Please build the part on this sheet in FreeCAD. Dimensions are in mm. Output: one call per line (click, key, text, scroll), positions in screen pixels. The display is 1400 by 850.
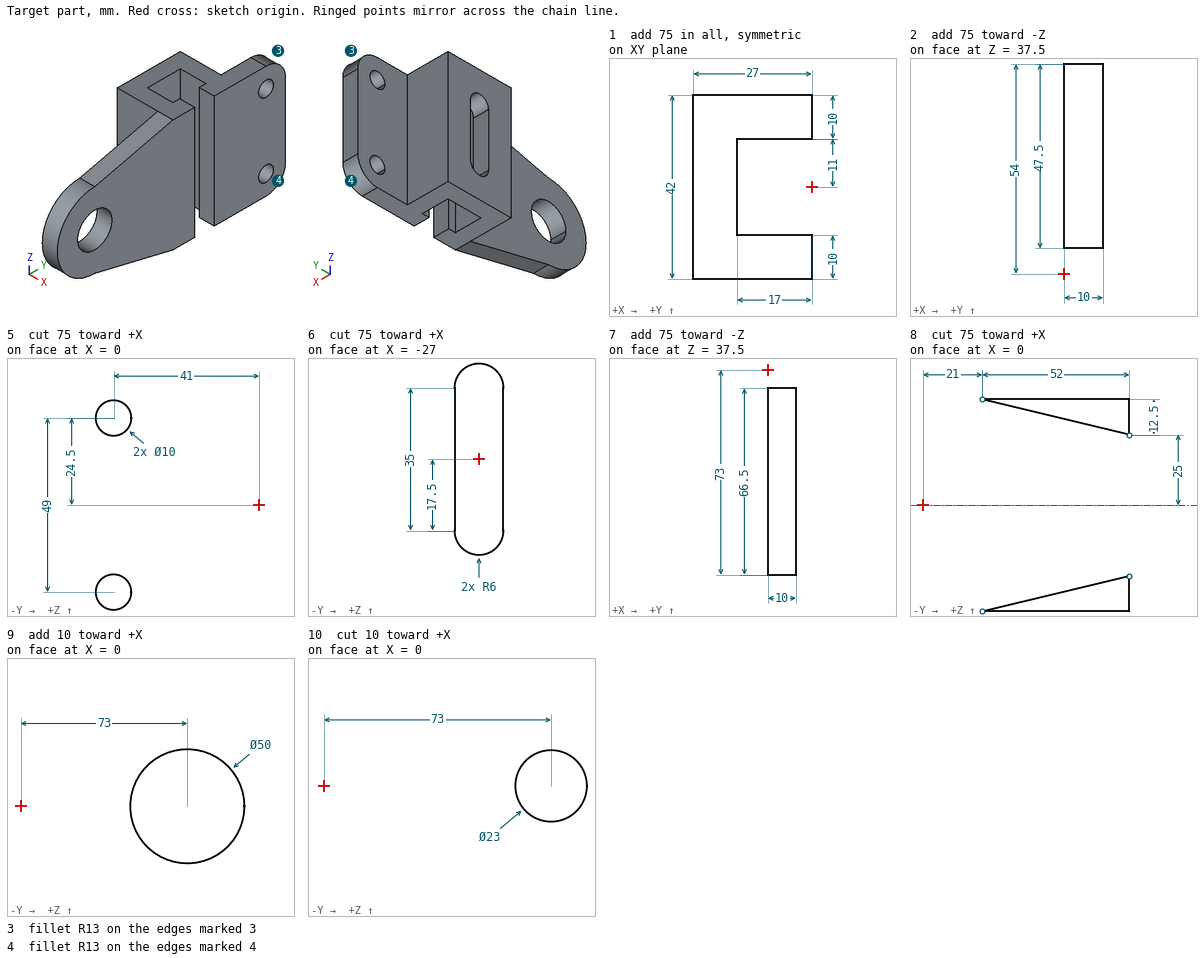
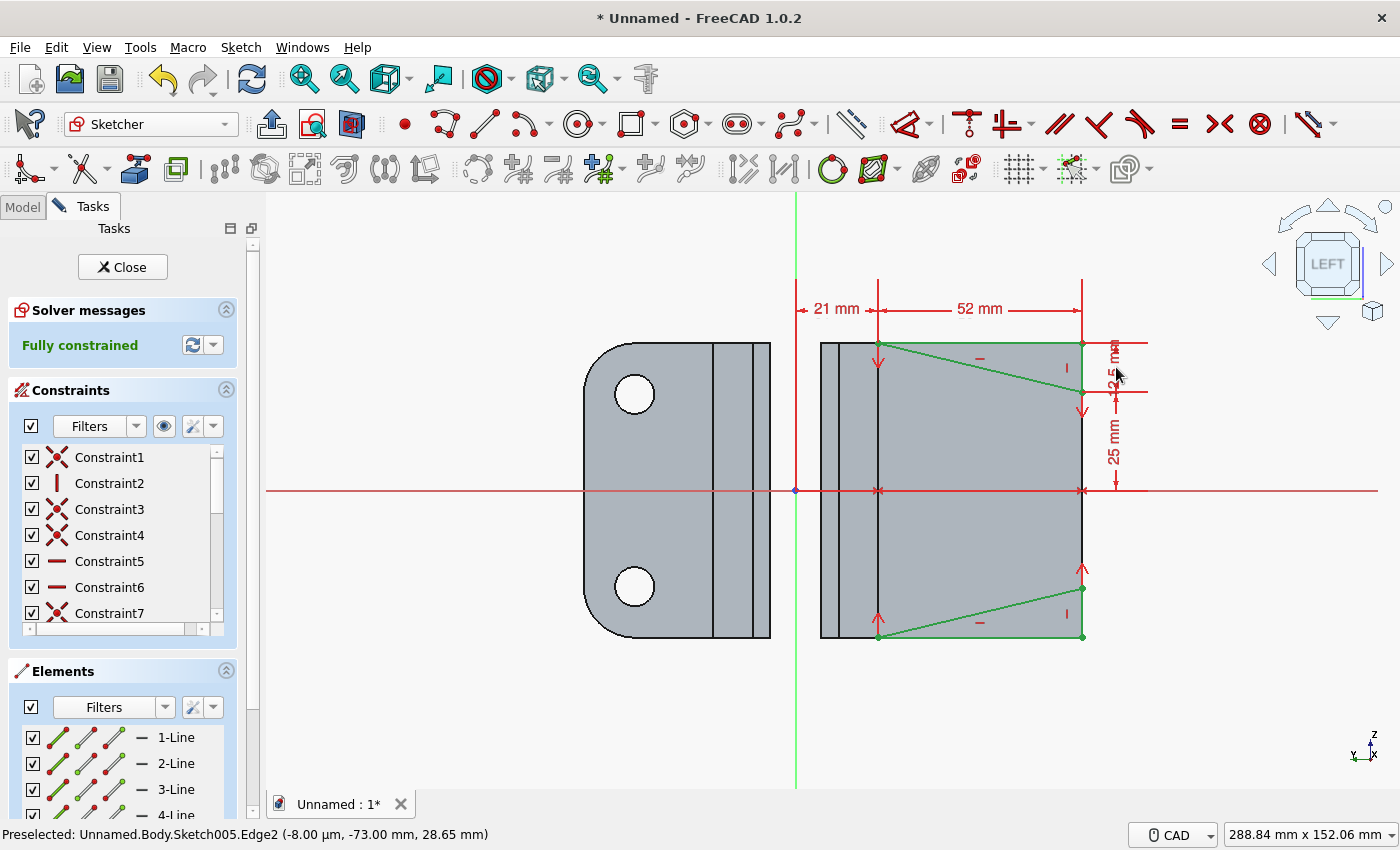
click(123, 267)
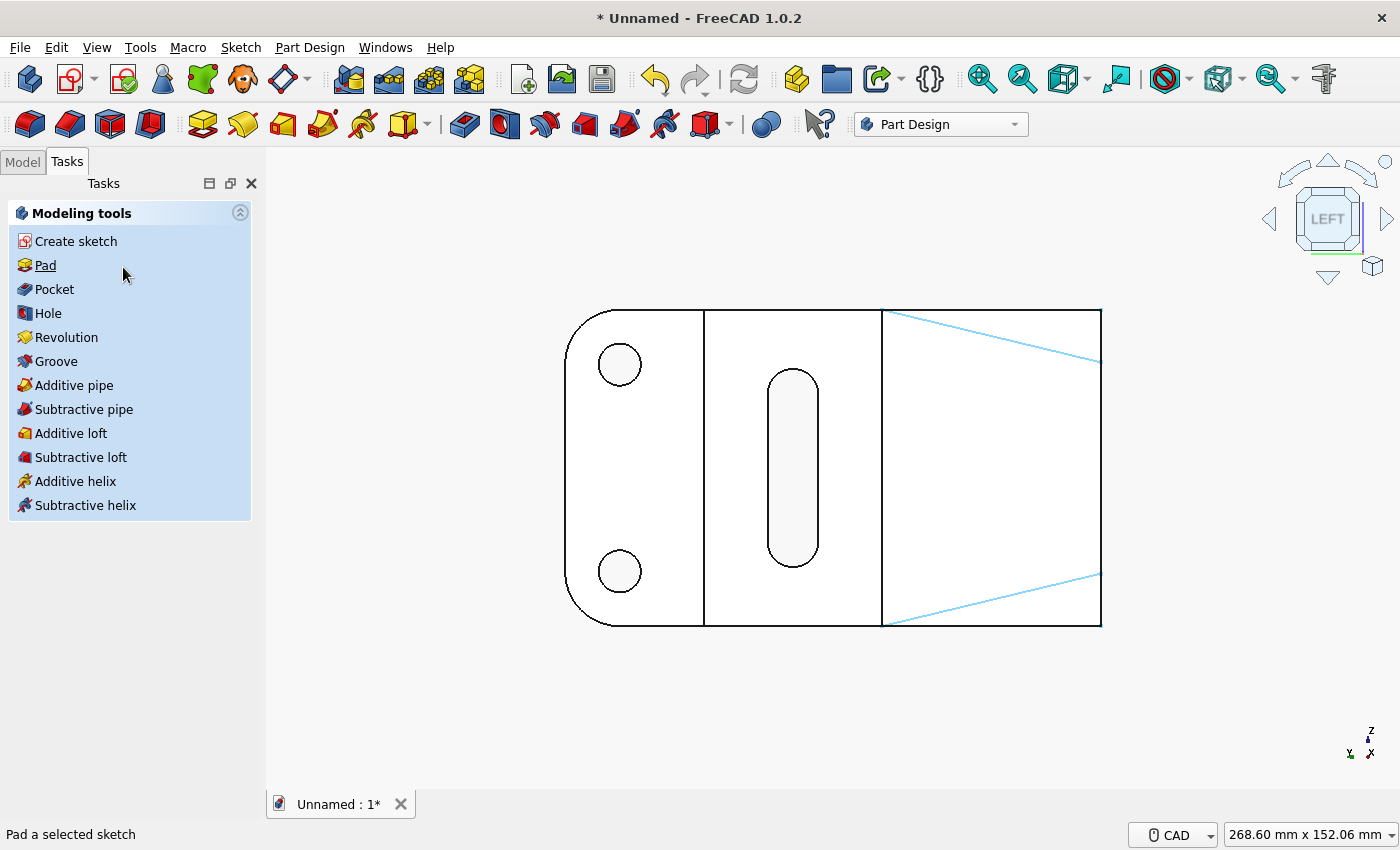
click(466, 124)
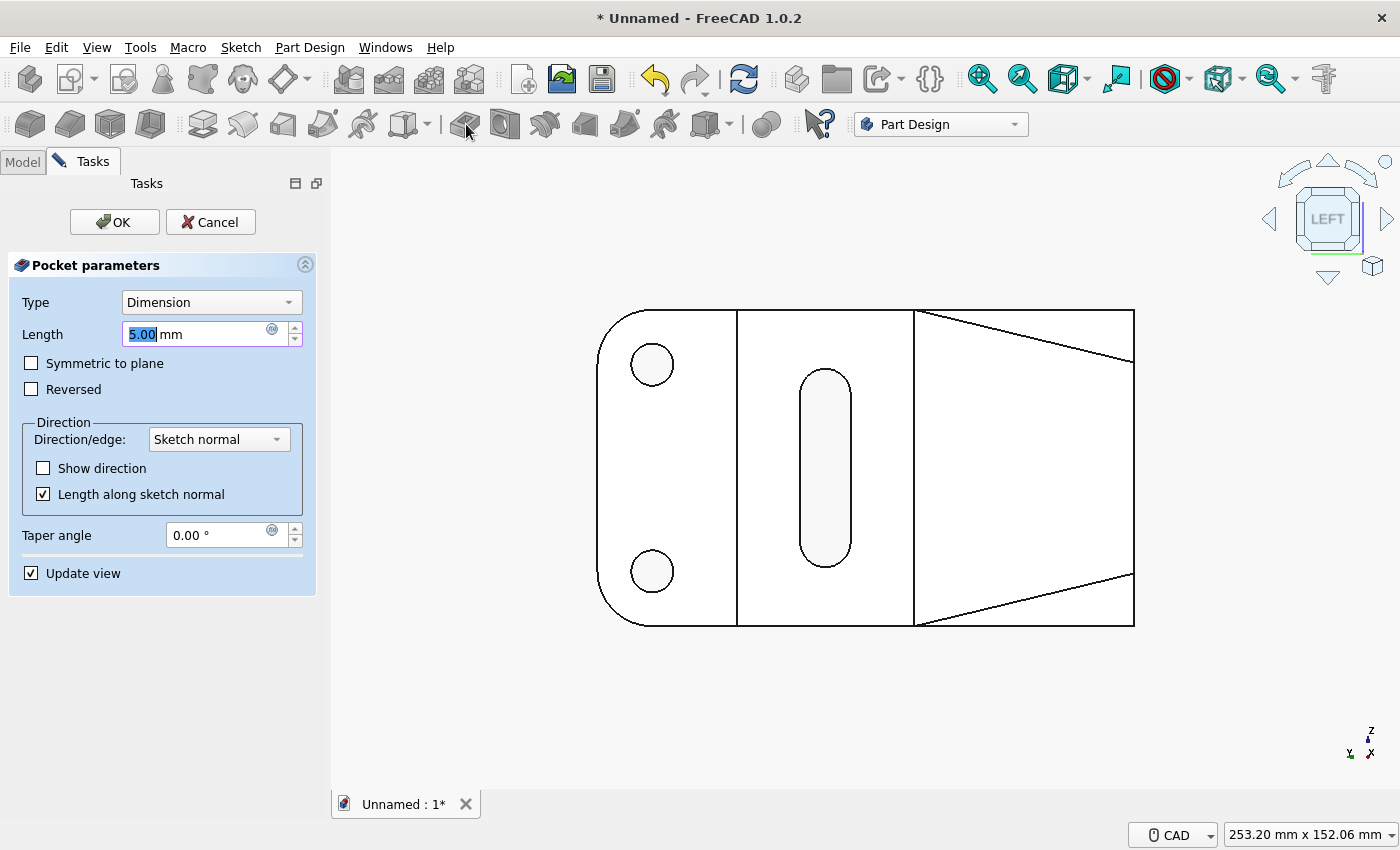
text(75)
key(Tab)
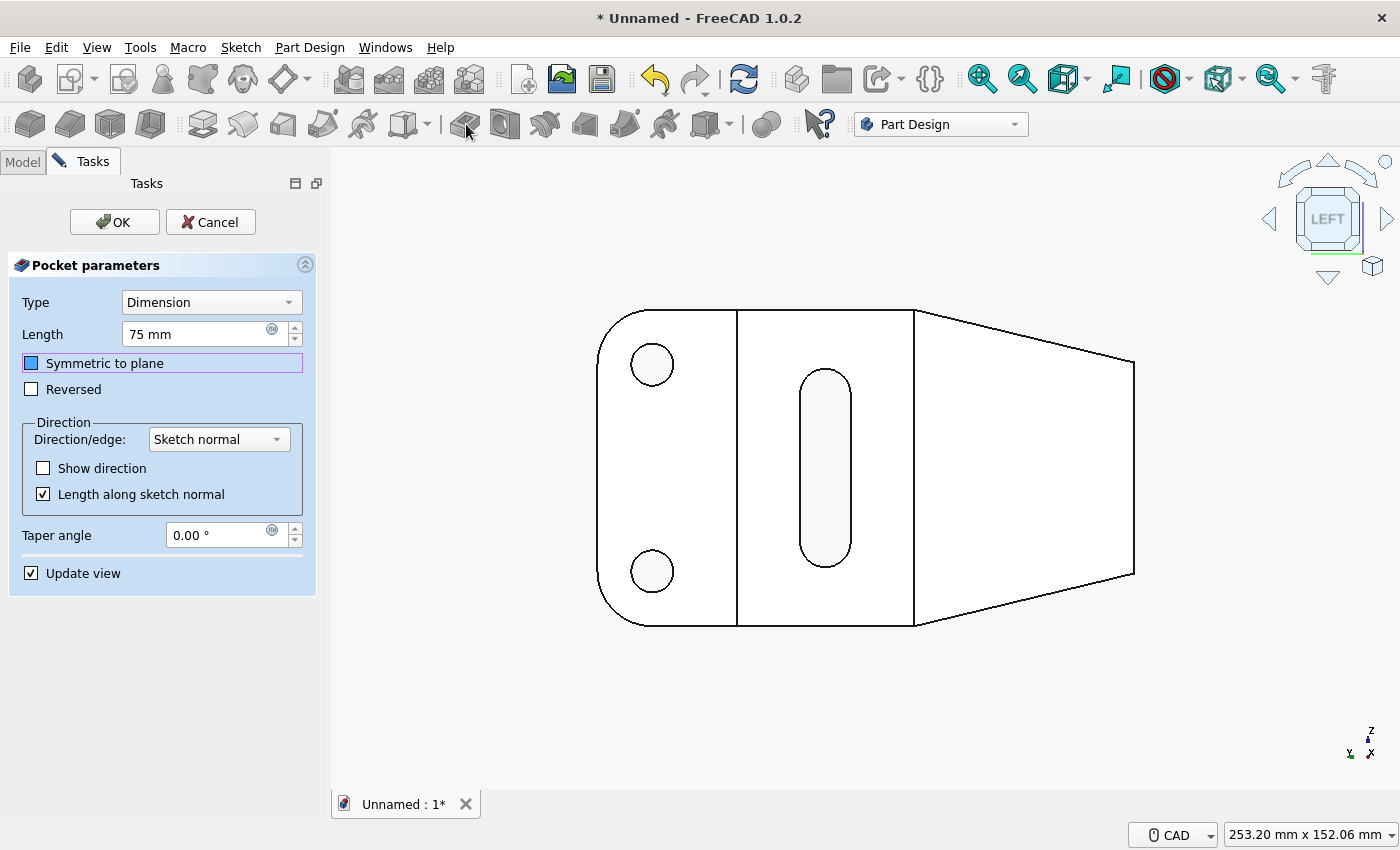
click(115, 222)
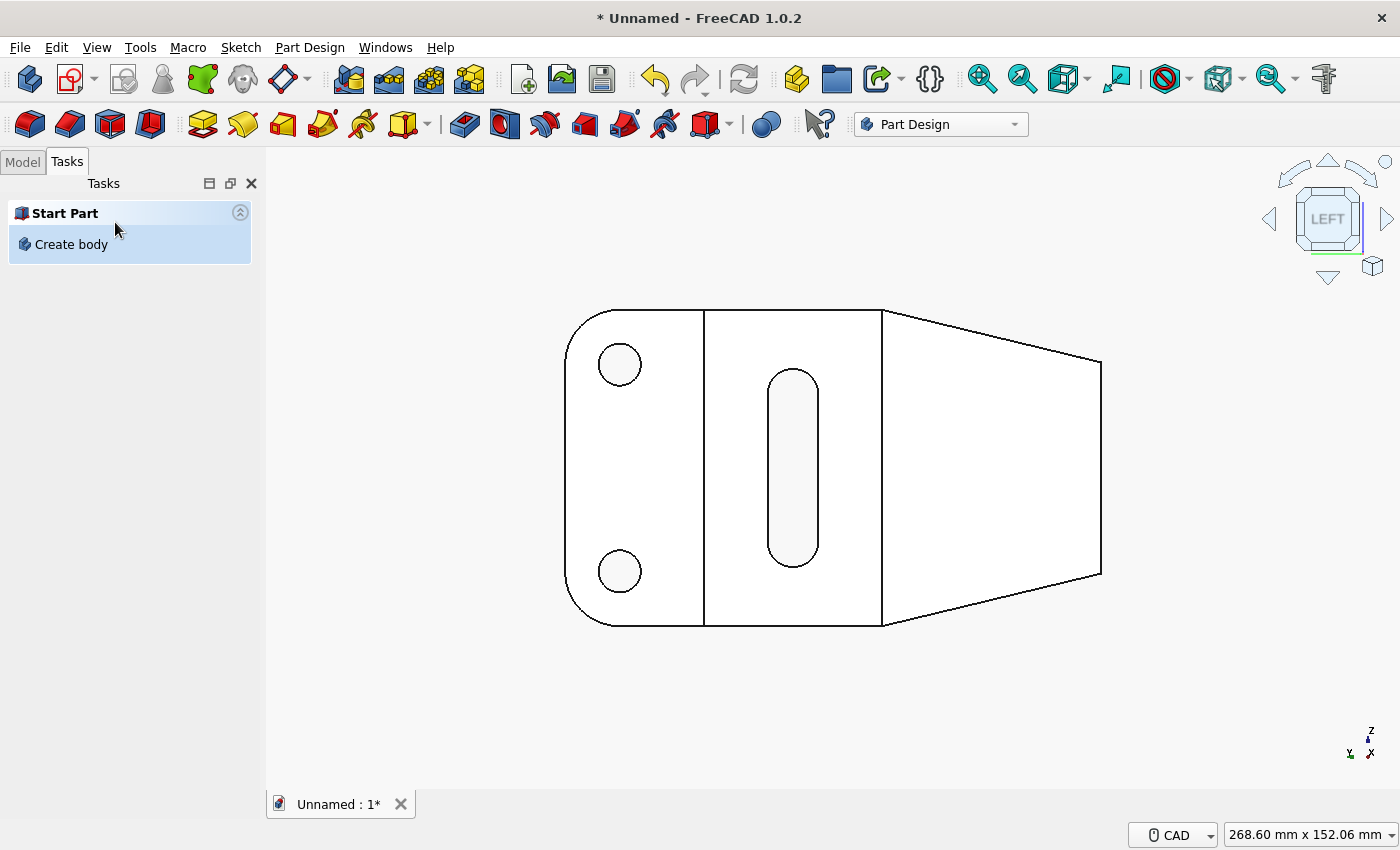
click(991, 467)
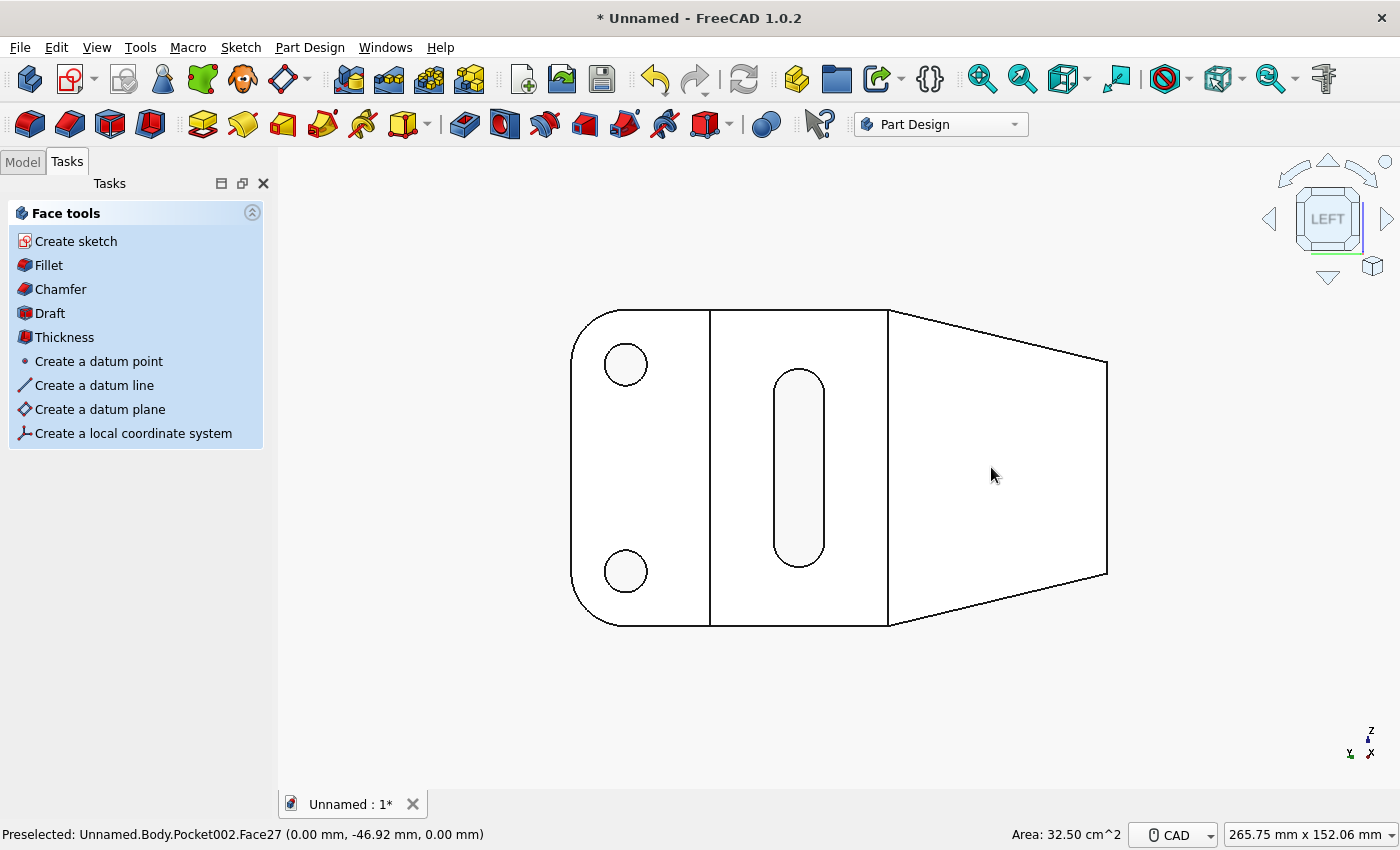
click(70, 80)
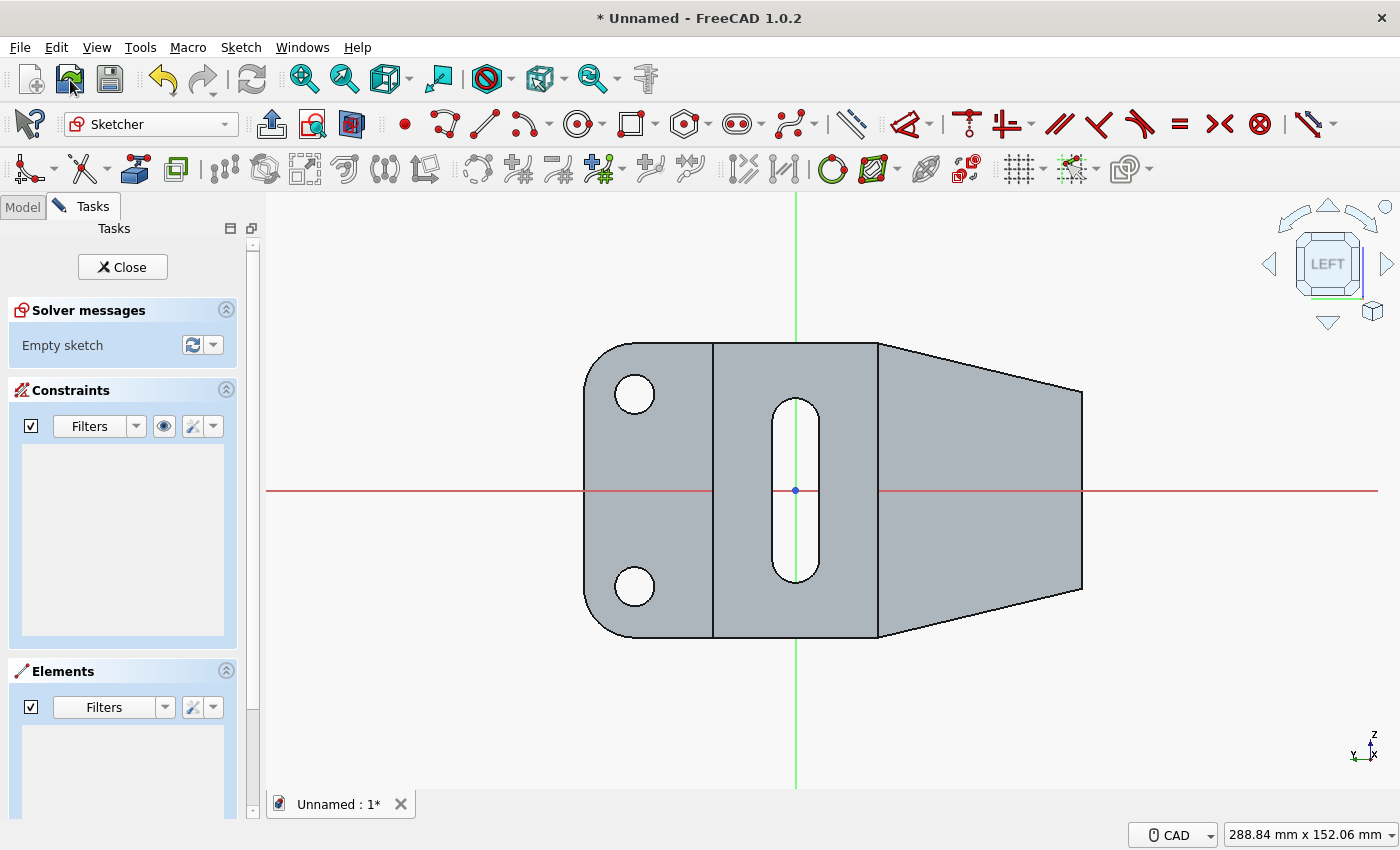
scroll(1235, 491, up, 3)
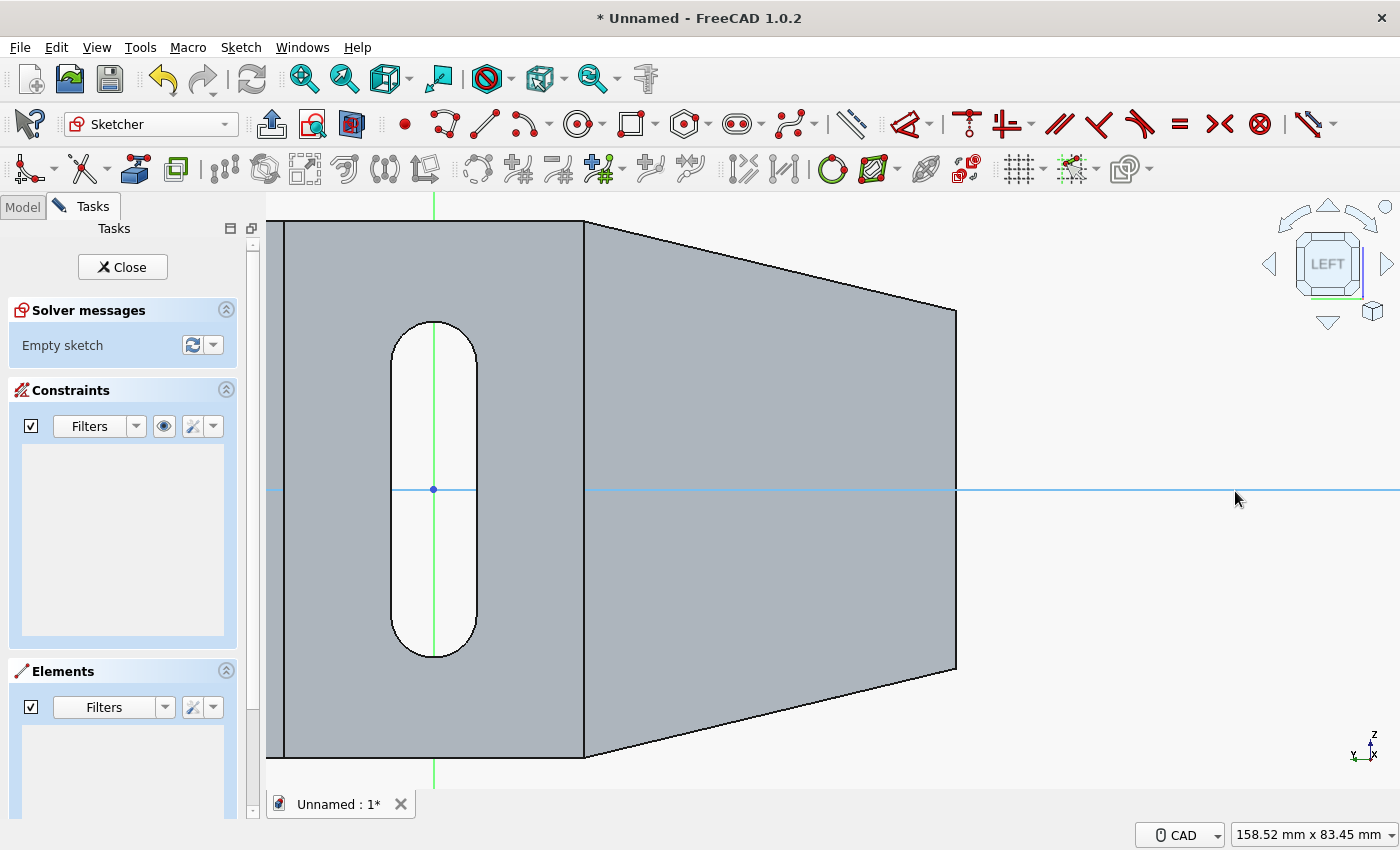
key(g)
key(c)